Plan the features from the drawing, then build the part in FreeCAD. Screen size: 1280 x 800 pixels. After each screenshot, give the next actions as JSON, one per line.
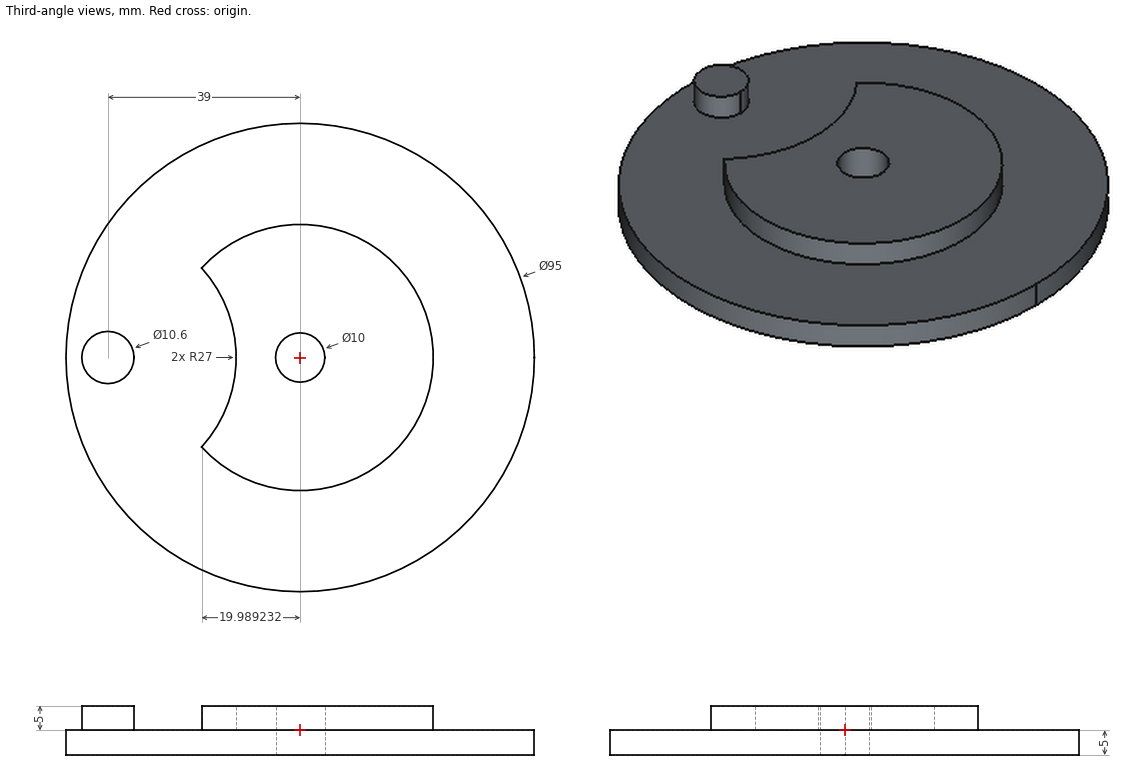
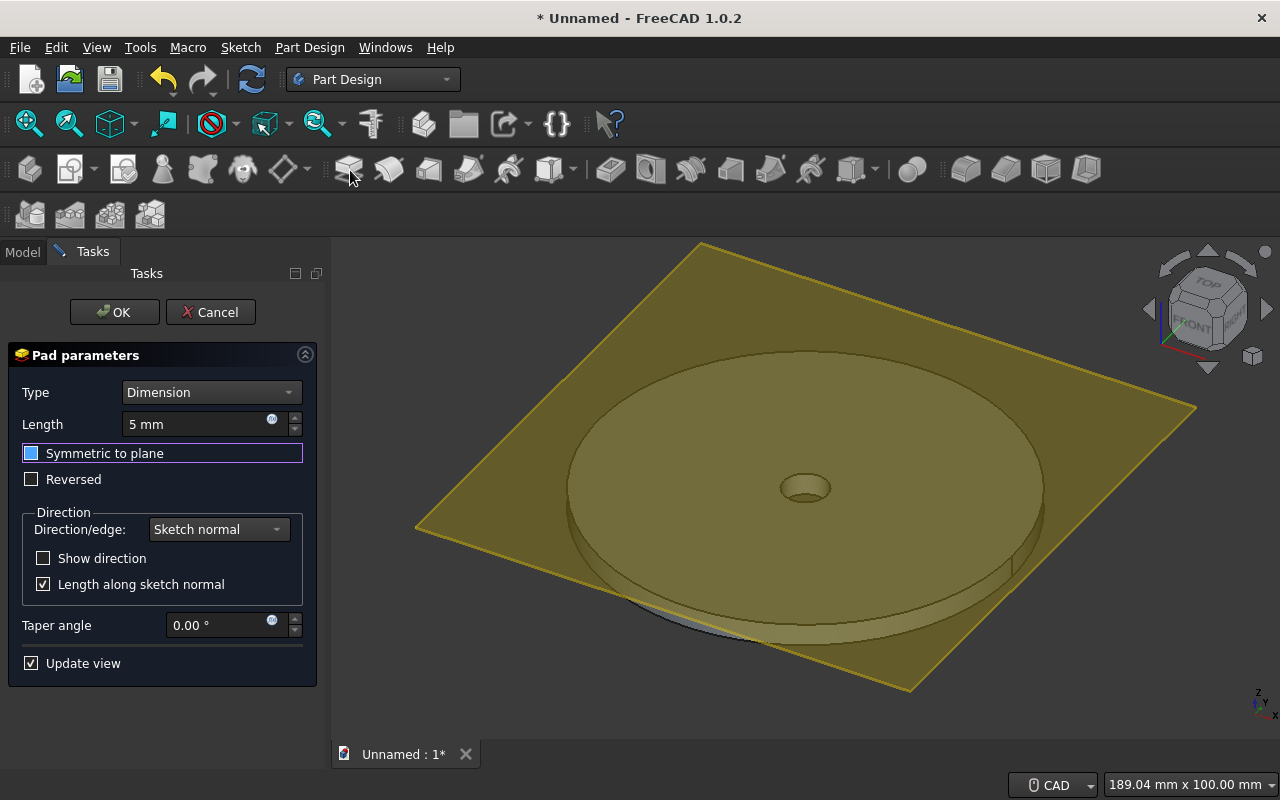
{"action": "left_click", "coordinate": [30, 479]}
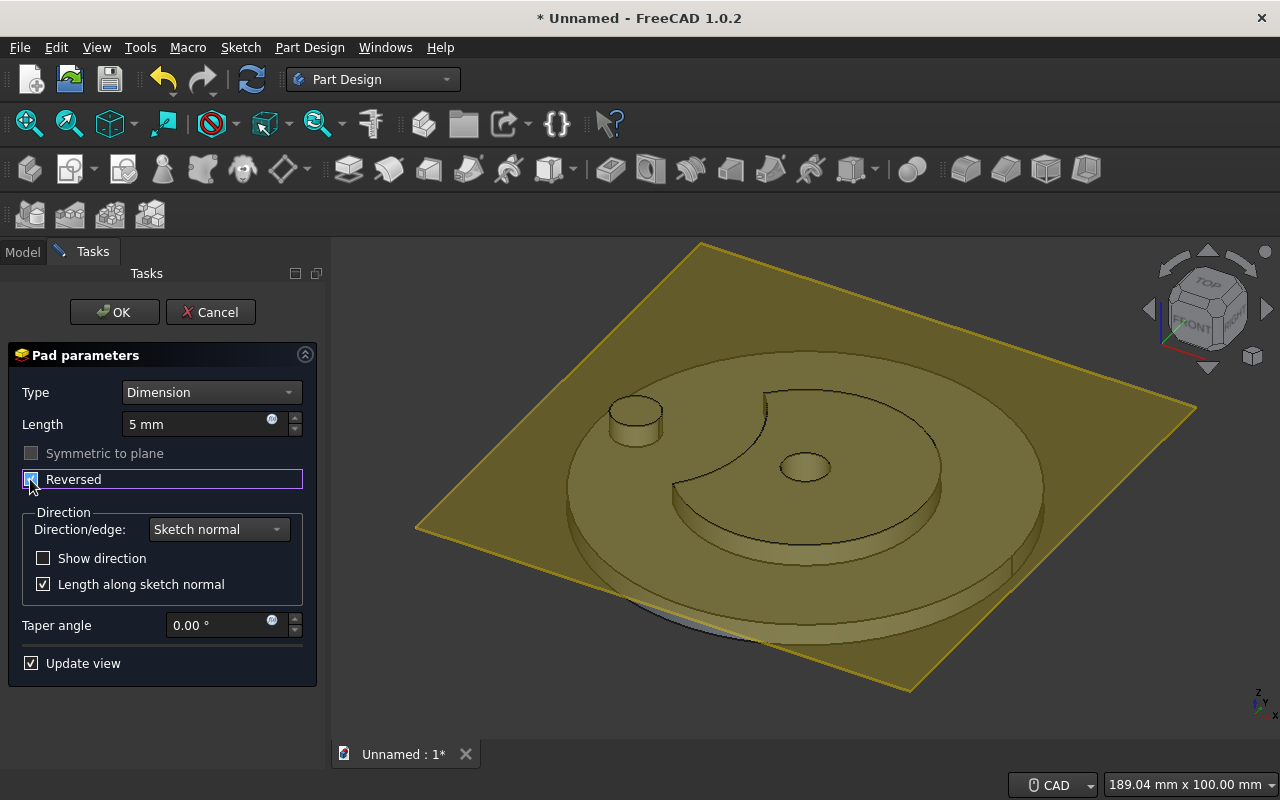
{"action": "left_click", "coordinate": [115, 312]}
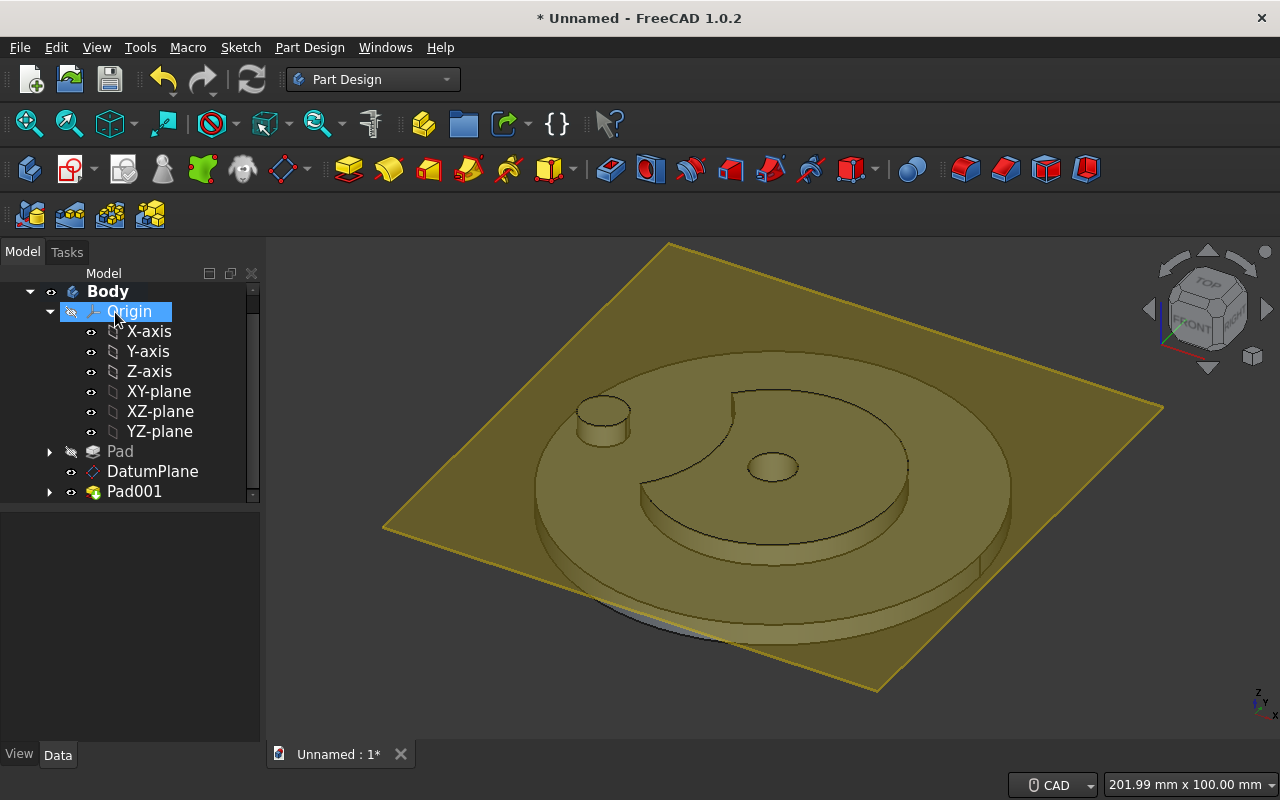
{"action": "left_click", "coordinate": [116, 472]}
{"action": "key", "text": "space"}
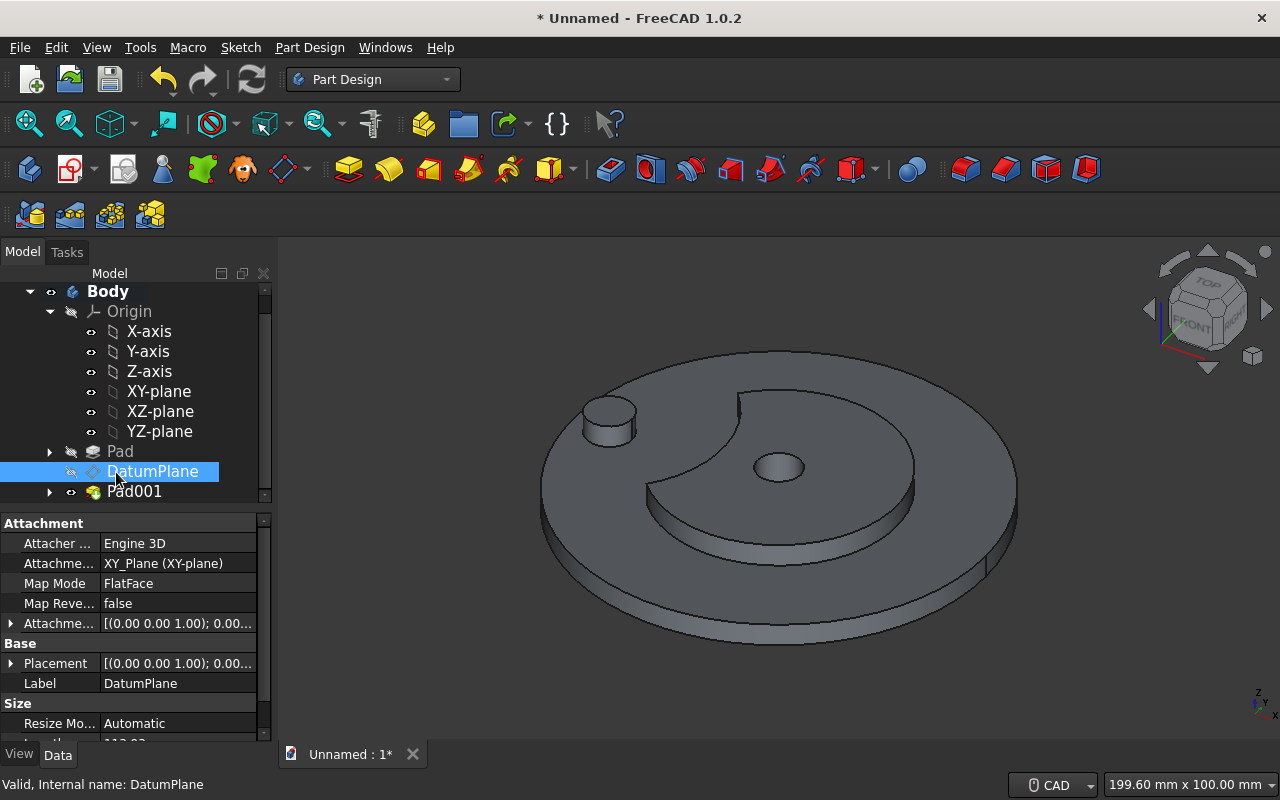
{"action": "key", "text": "0"}